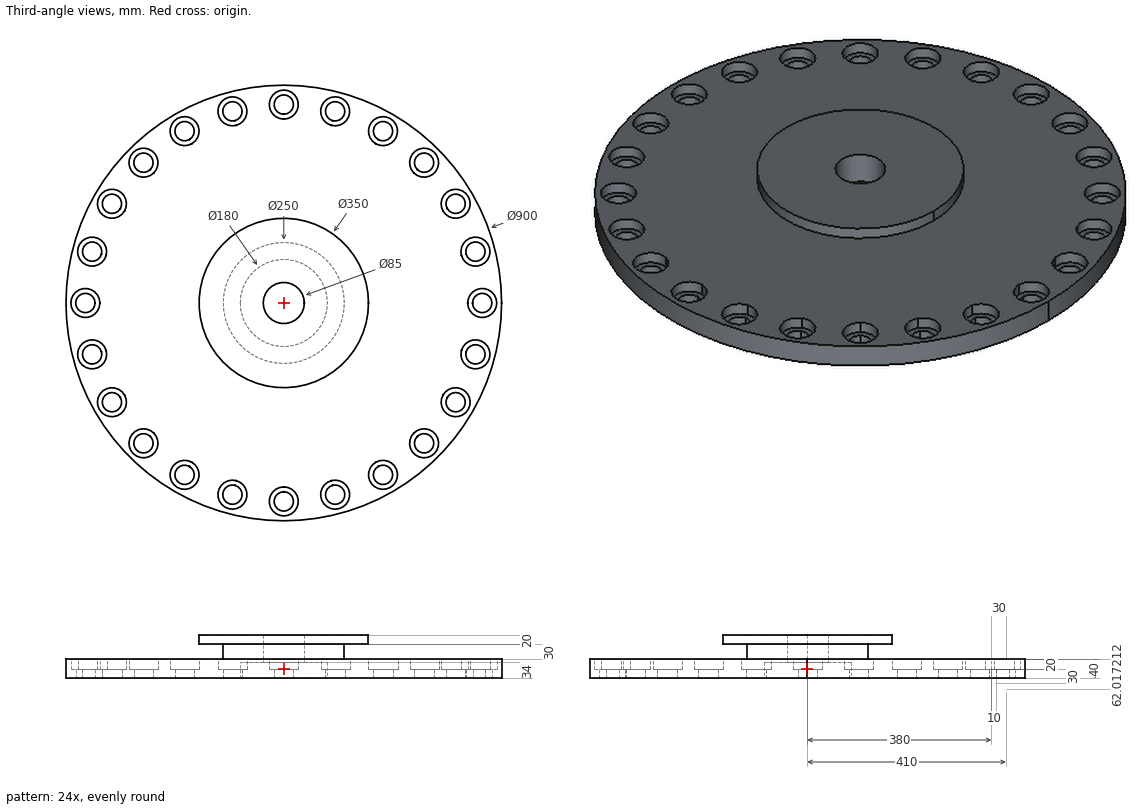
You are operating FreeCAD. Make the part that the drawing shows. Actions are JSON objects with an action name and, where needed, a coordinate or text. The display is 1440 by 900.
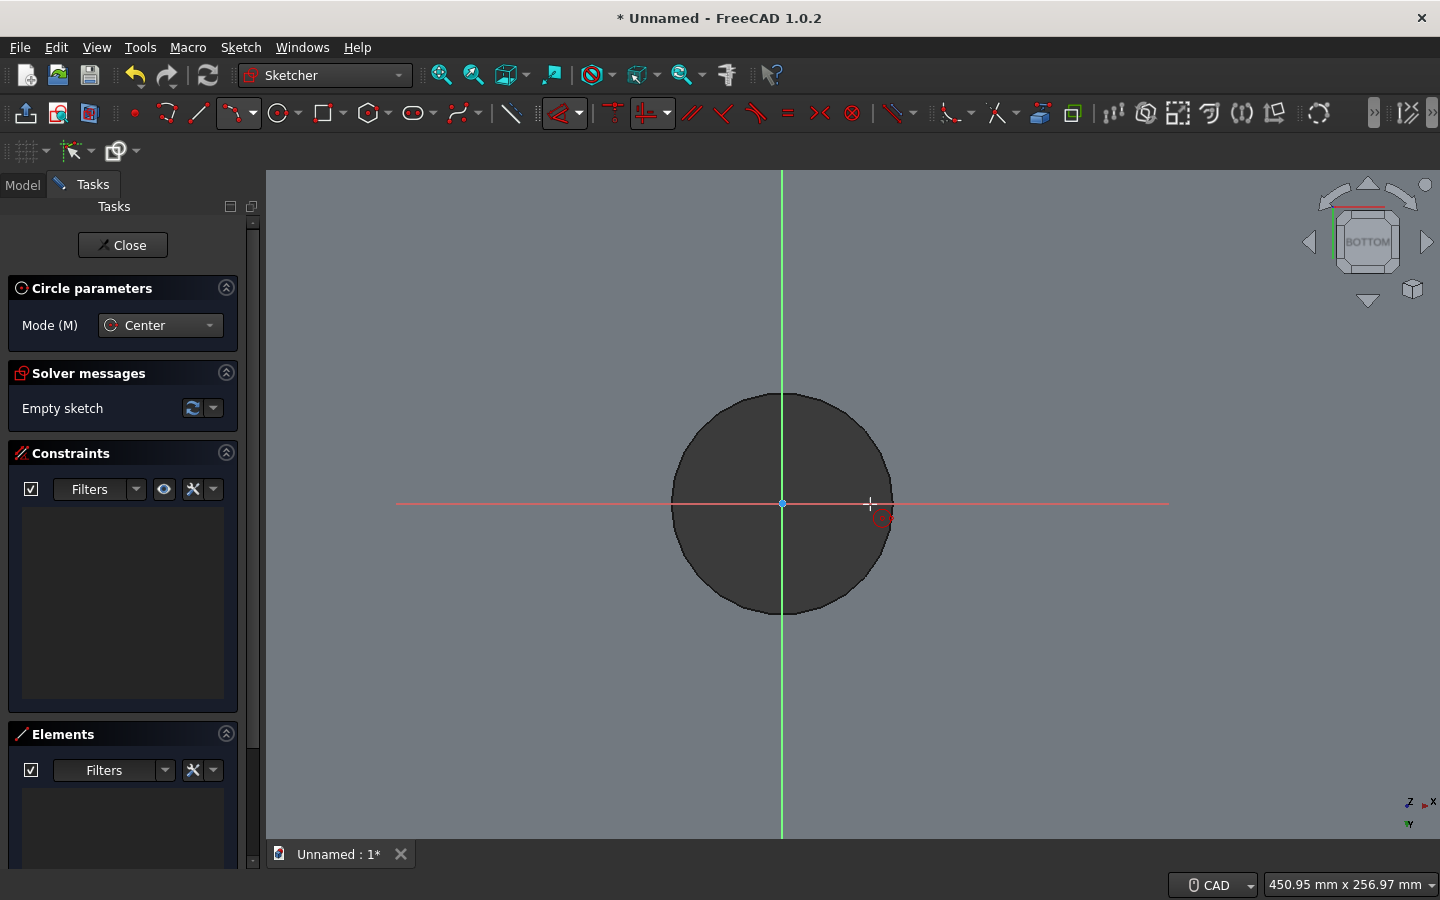
{"action": "left_click", "coordinate": [782, 504]}
{"action": "mouse_move", "coordinate": [948, 338]}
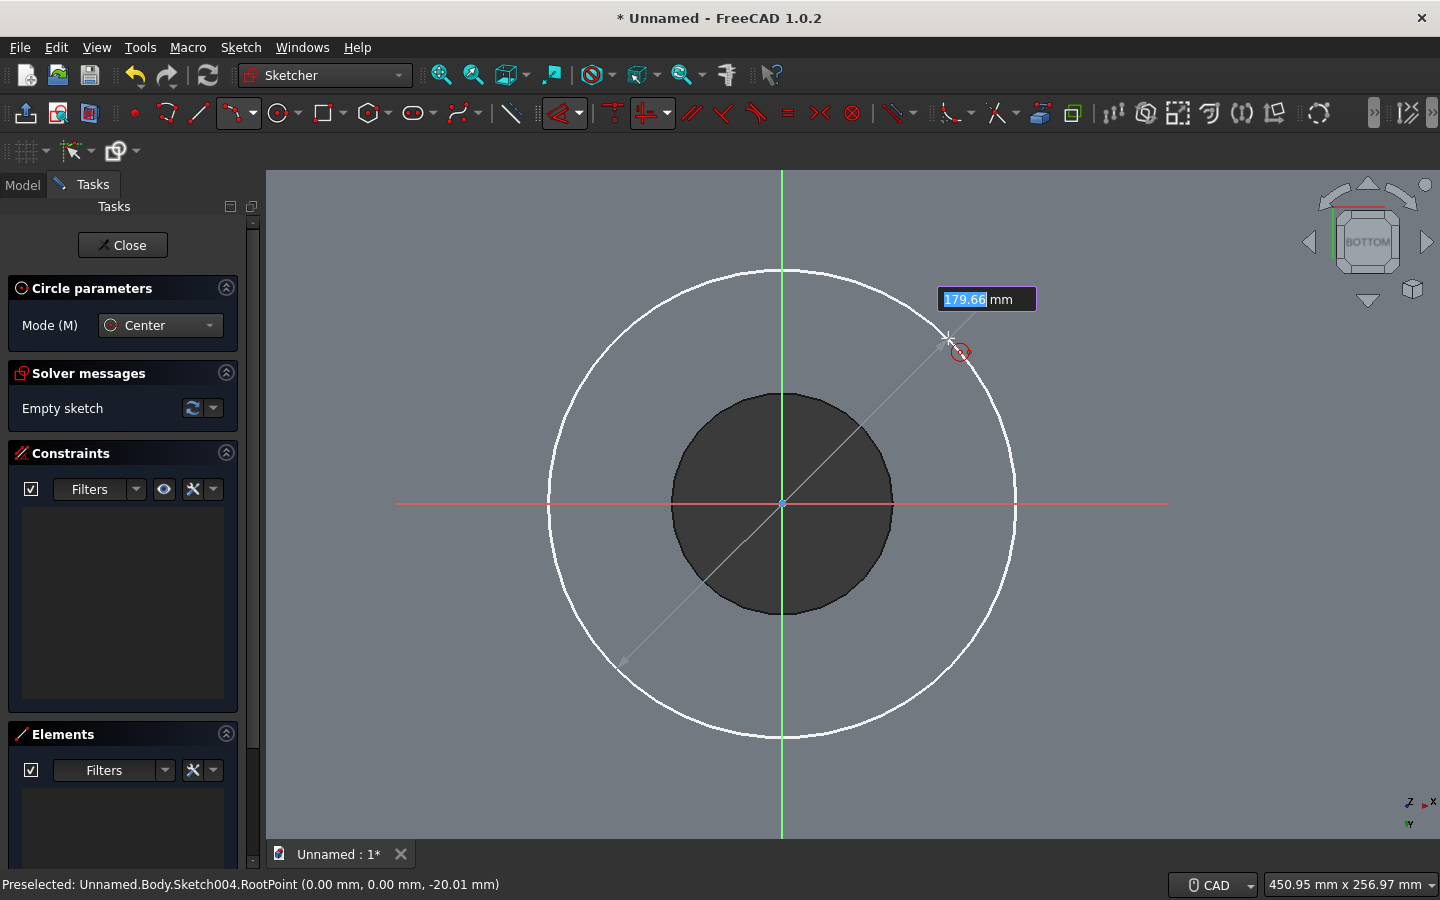
{"action": "type", "text": "180"}
{"action": "key", "text": "Return"}
{"action": "key", "text": "Escape"}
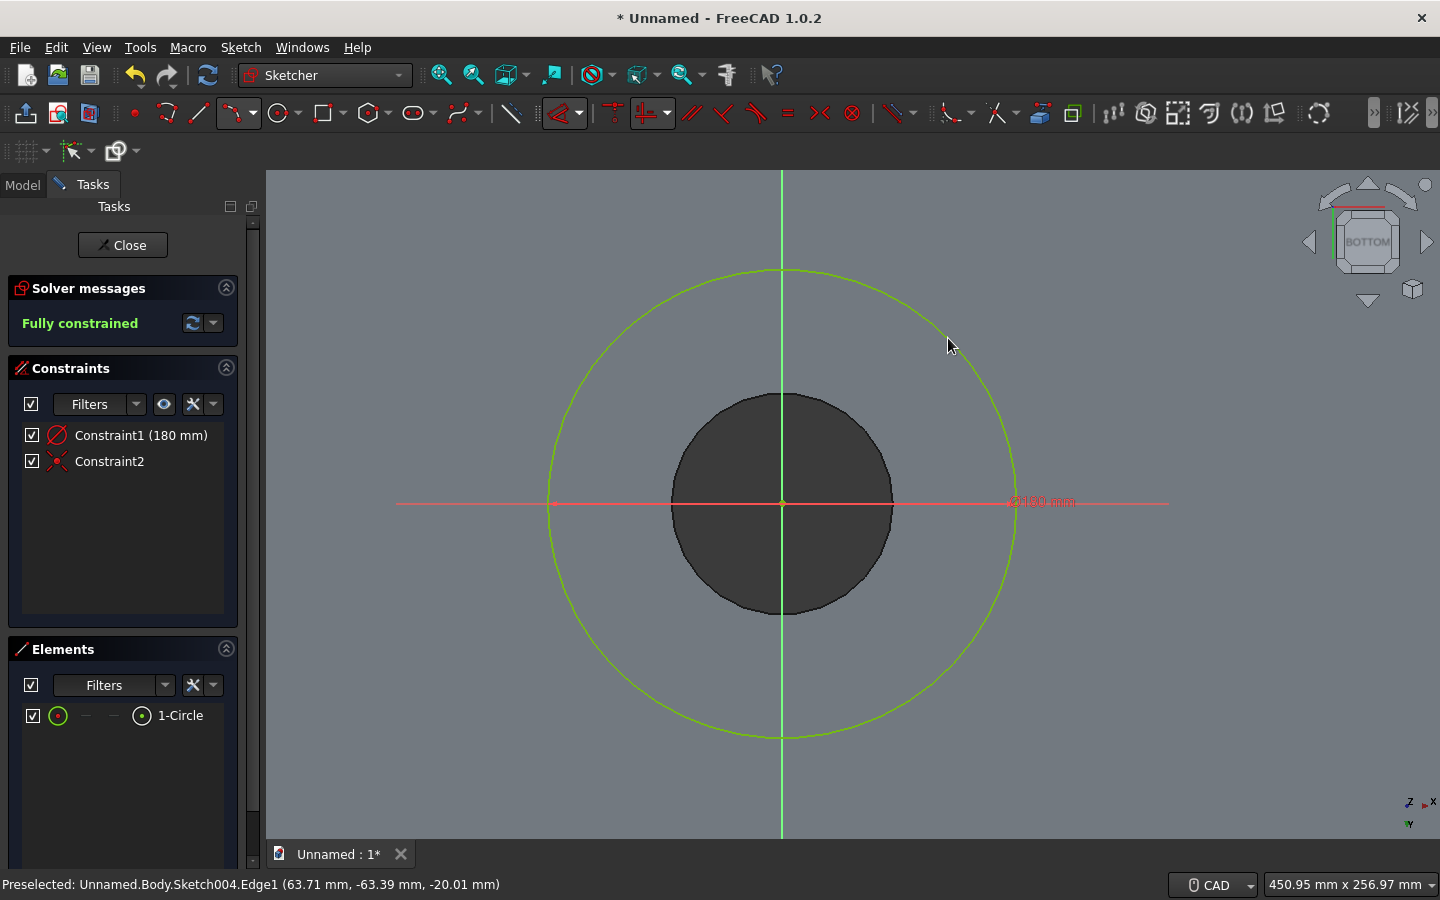
{"action": "left_click", "coordinate": [123, 245]}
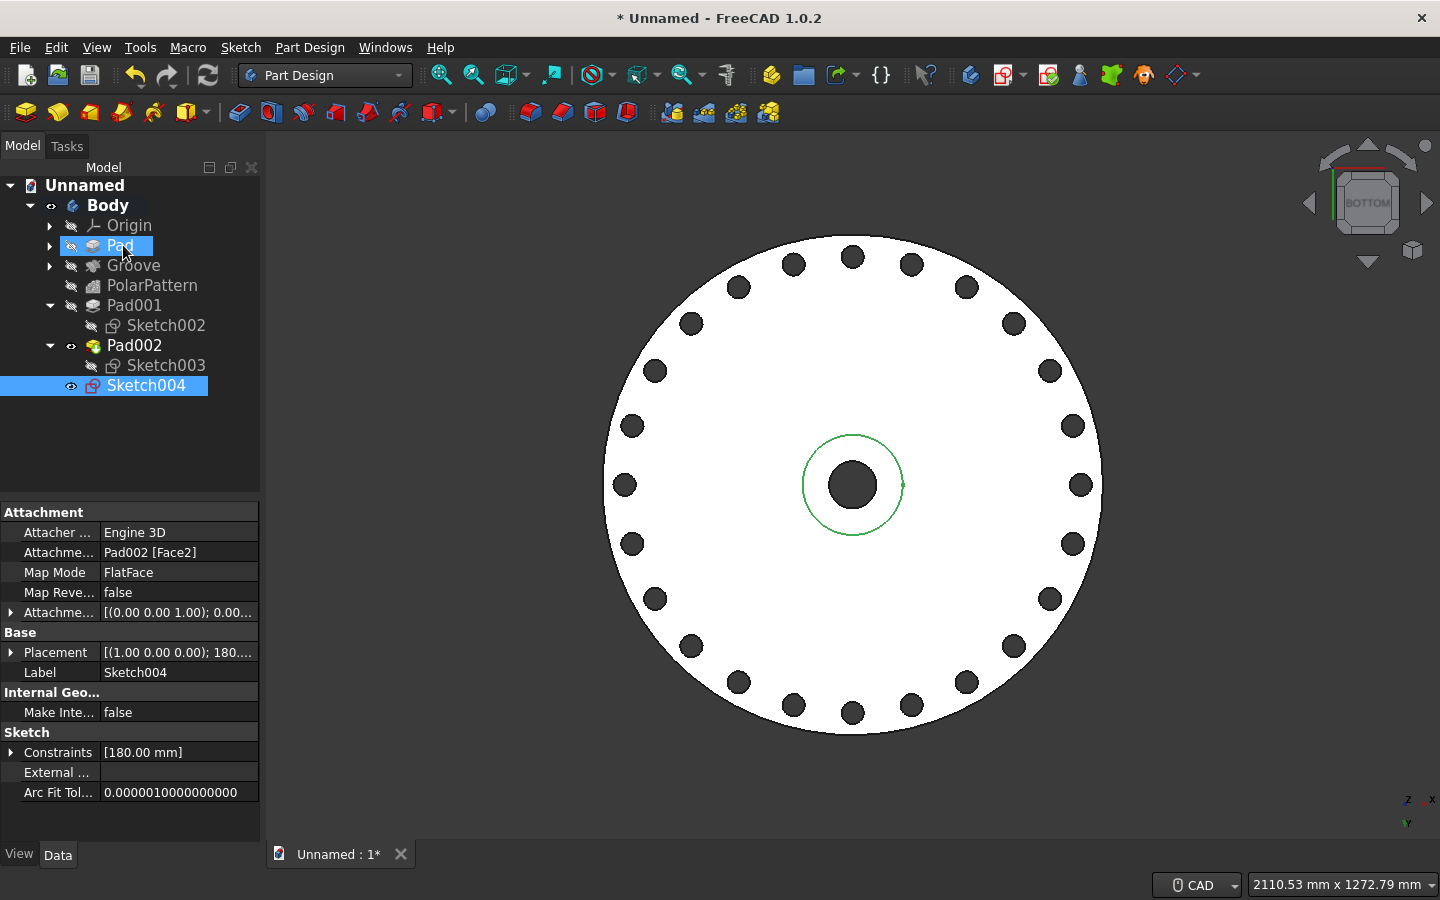
{"action": "left_click", "coordinate": [240, 112]}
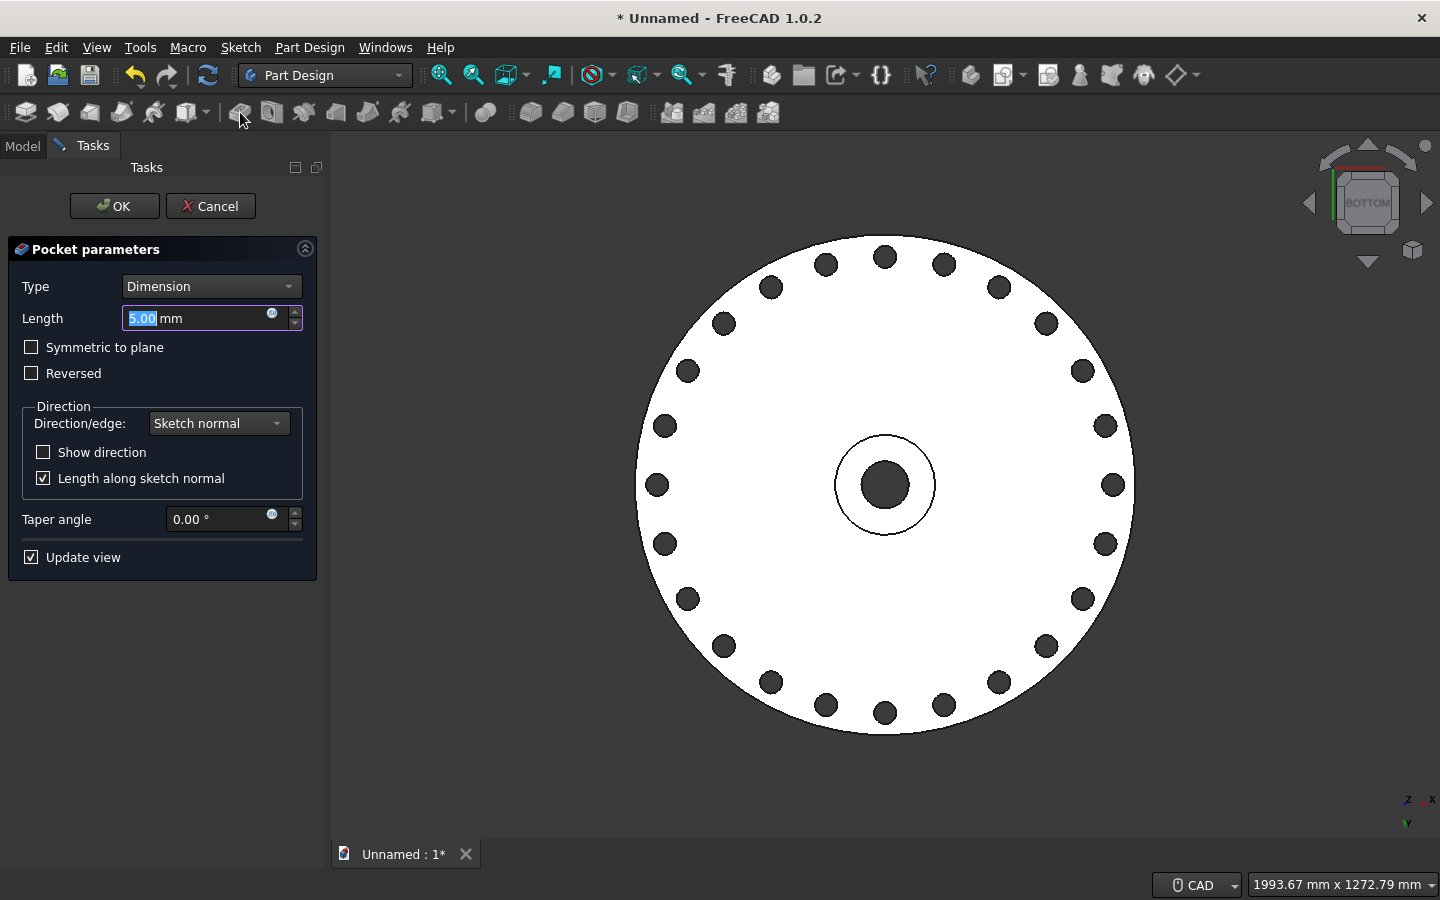
{"action": "type", "text": "34"}
{"action": "key", "text": "Tab"}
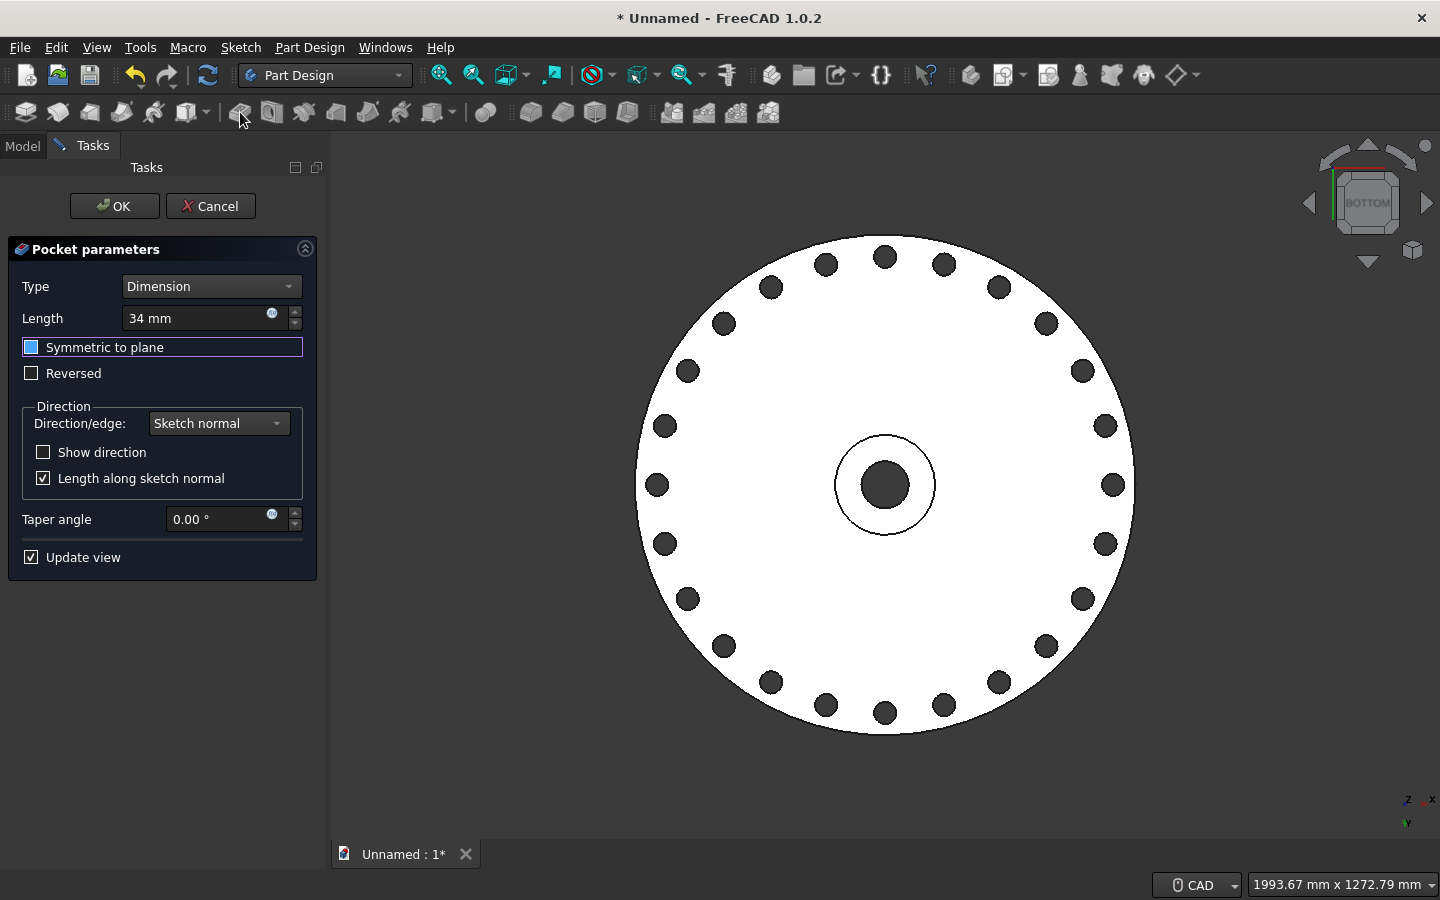
{"action": "left_click", "coordinate": [115, 206]}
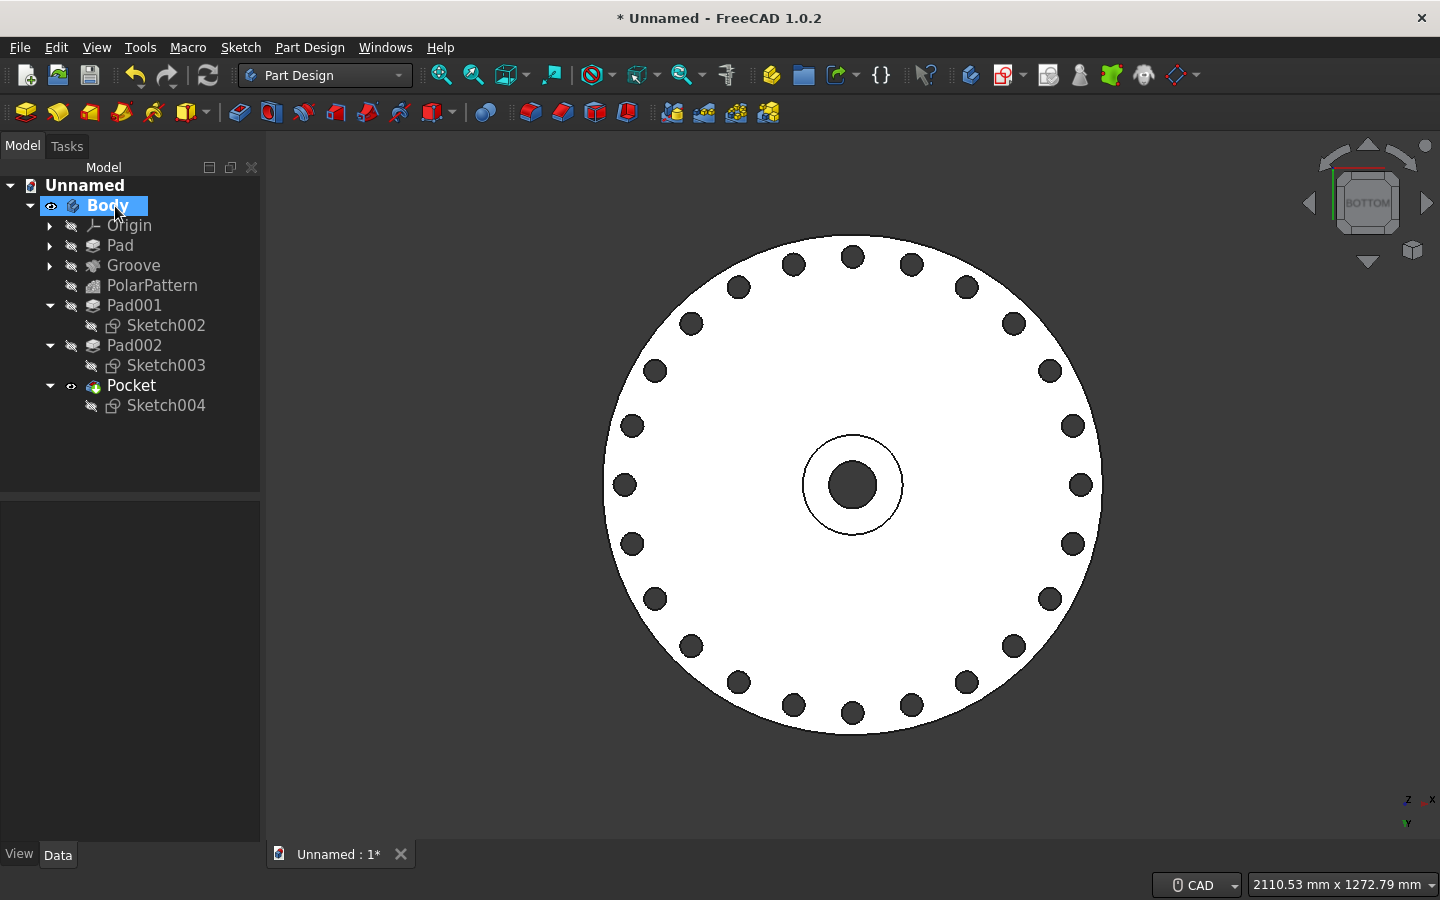
{"action": "key", "text": "0"}